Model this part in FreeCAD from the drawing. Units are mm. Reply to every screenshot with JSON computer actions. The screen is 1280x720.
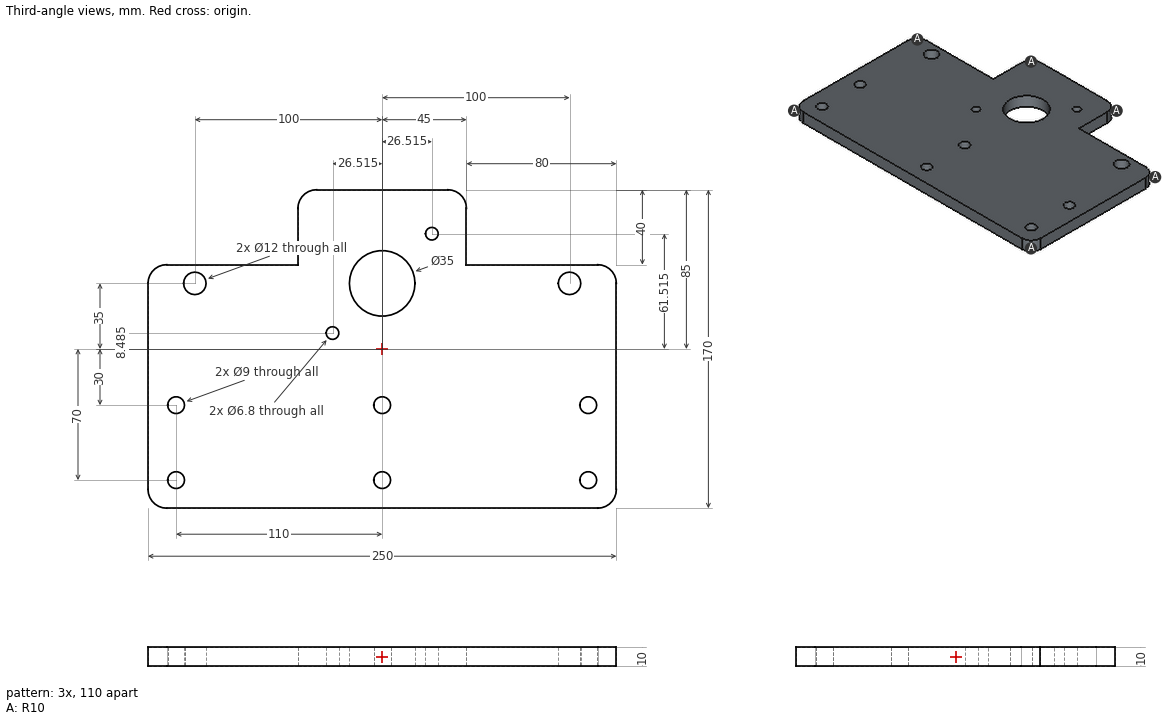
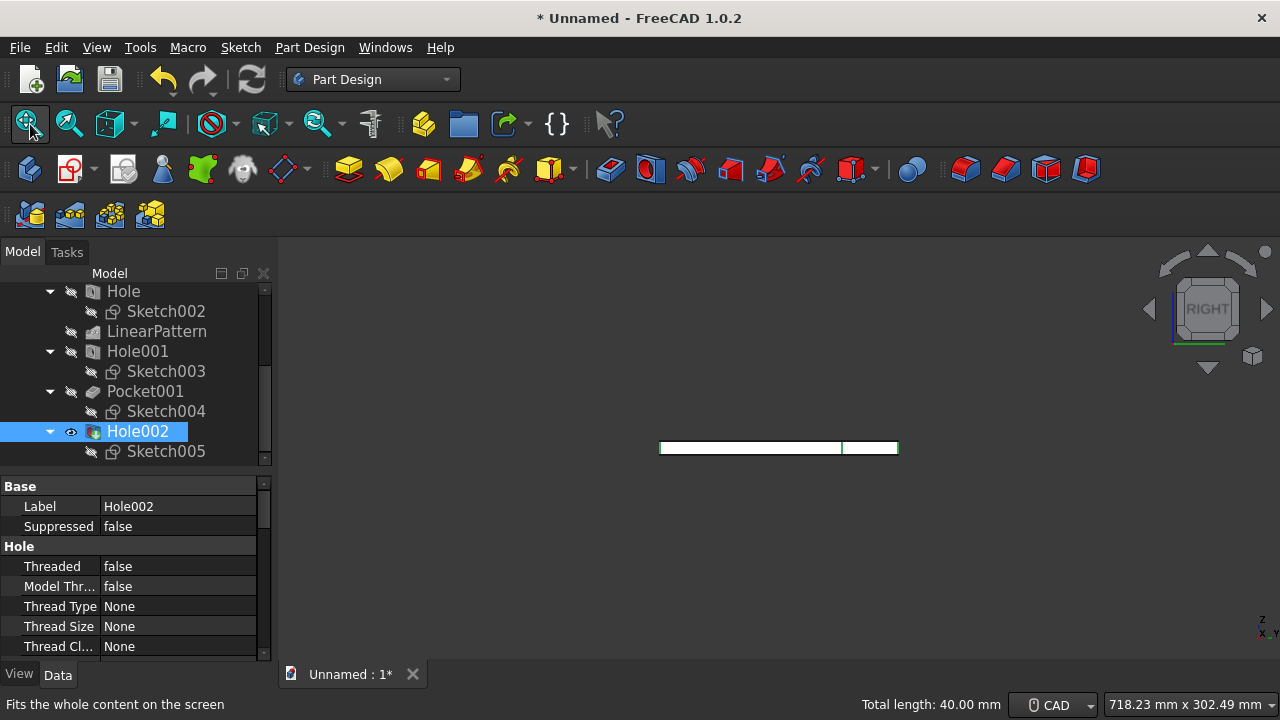
{"action": "key", "text": "5"}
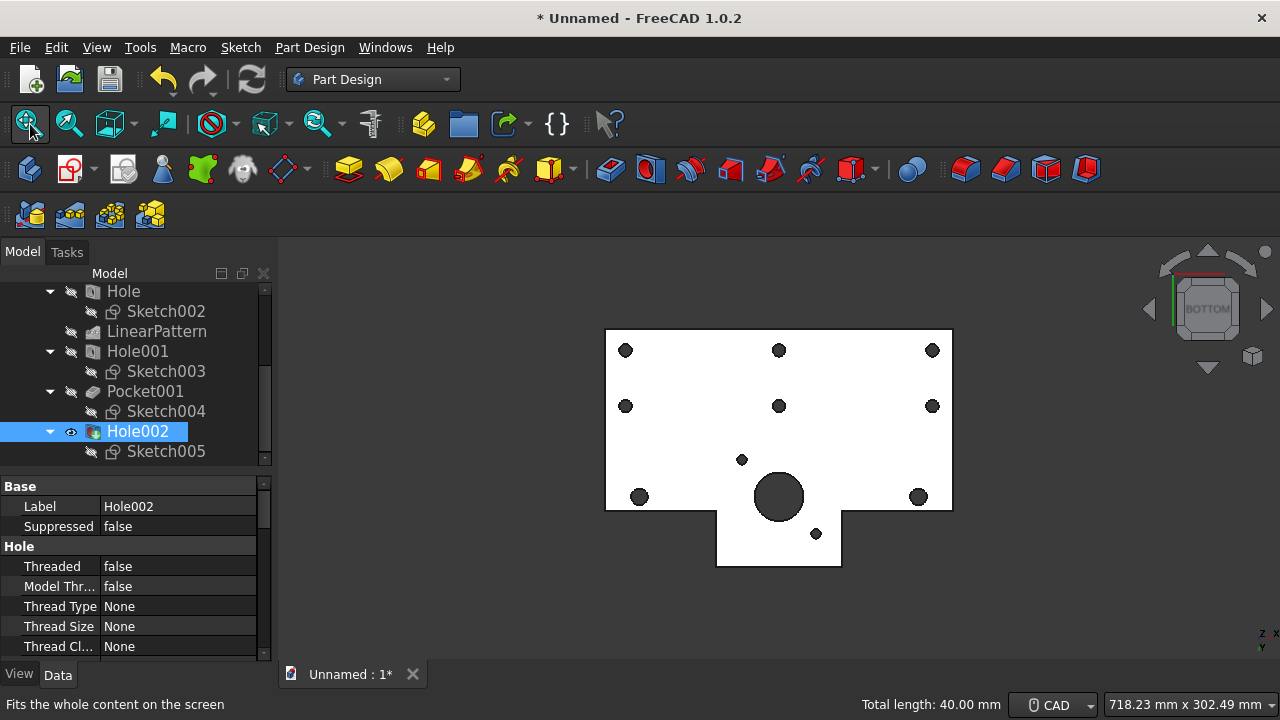
{"action": "scroll", "coordinate": [716, 566], "scroll_direction": "up", "scroll_amount": 6}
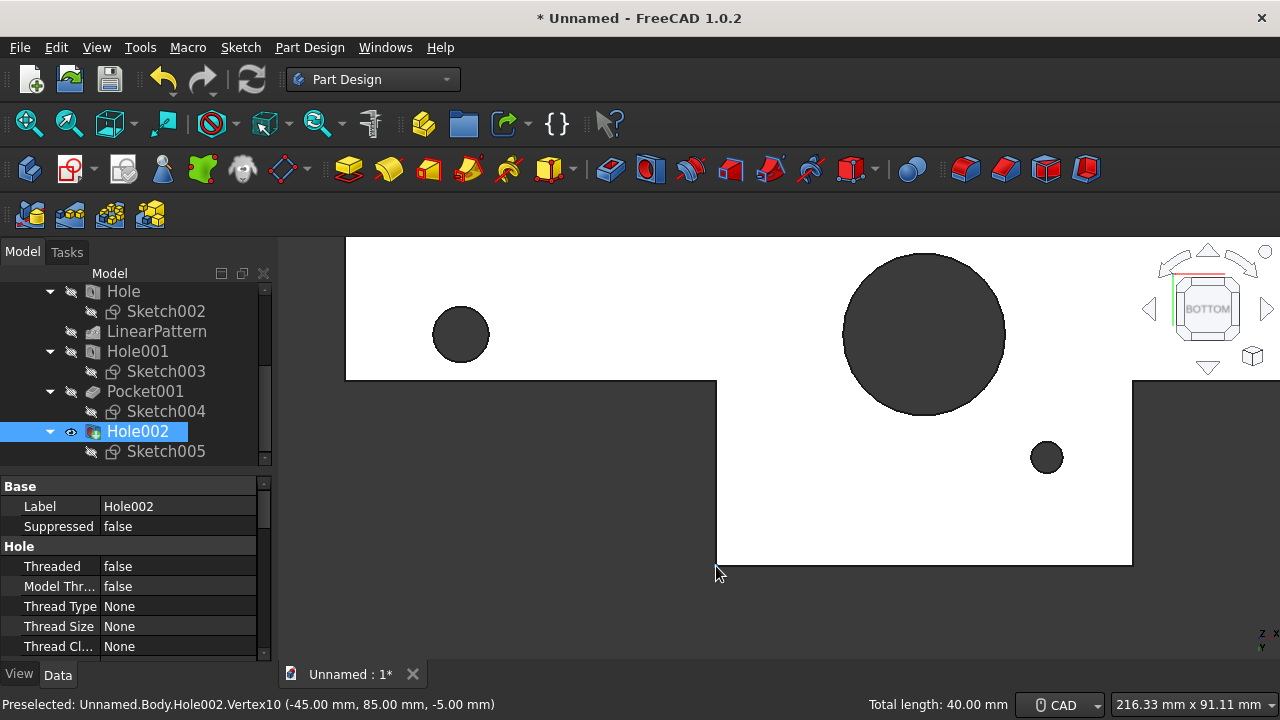
{"action": "left_click", "coordinate": [30, 124]}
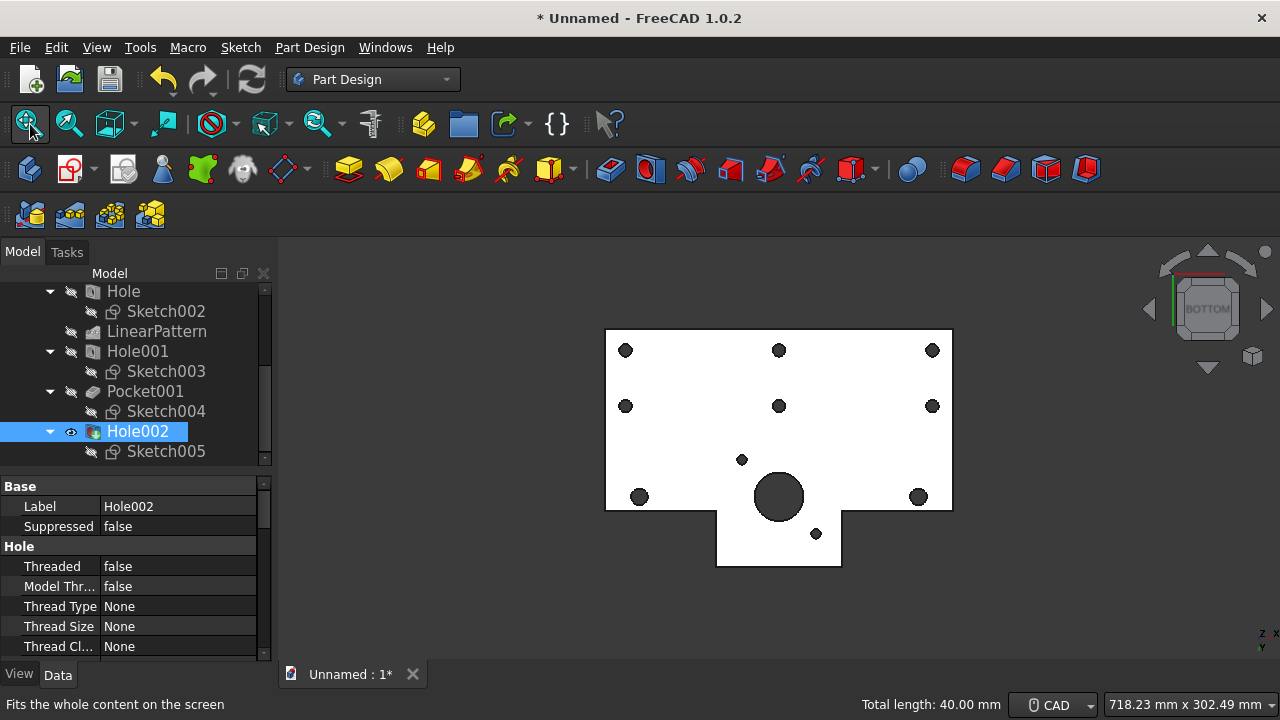
{"action": "key", "text": "4"}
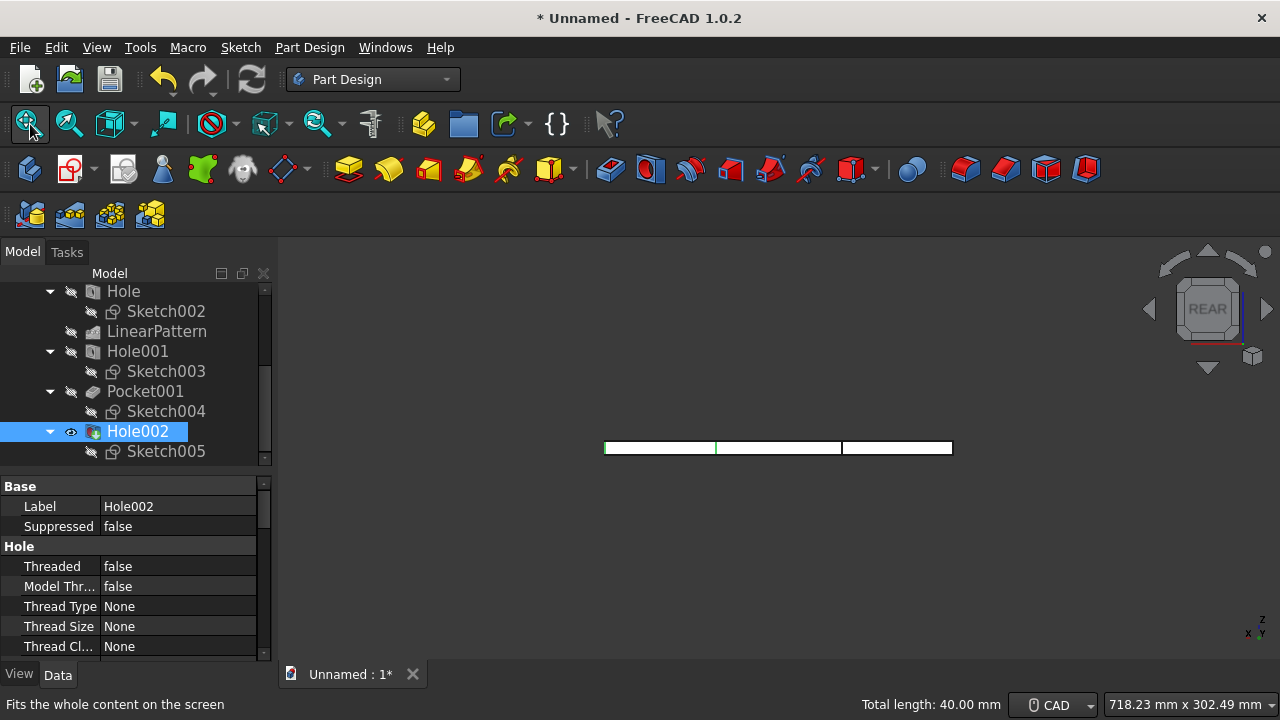
{"action": "left_click", "coordinate": [30, 124]}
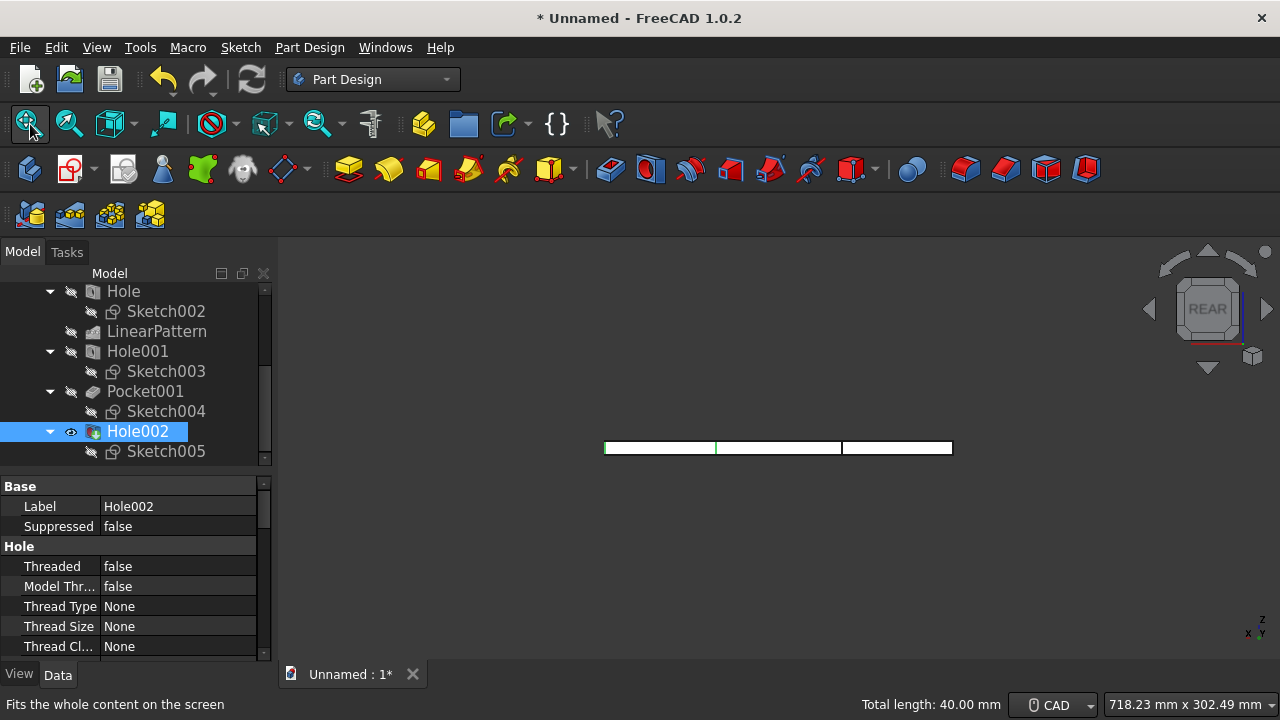
{"action": "left_click", "coordinate": [842, 447], "text": "ctrl"}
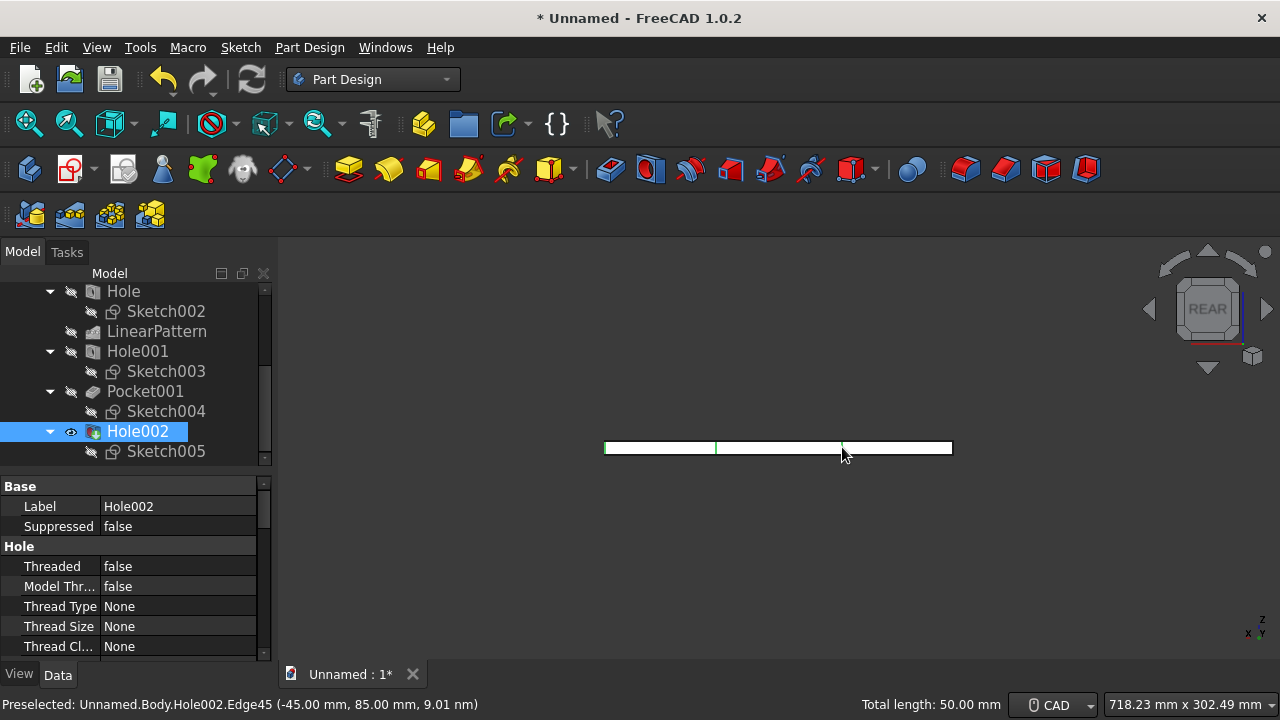
{"action": "left_click", "coordinate": [953, 447], "text": "ctrl"}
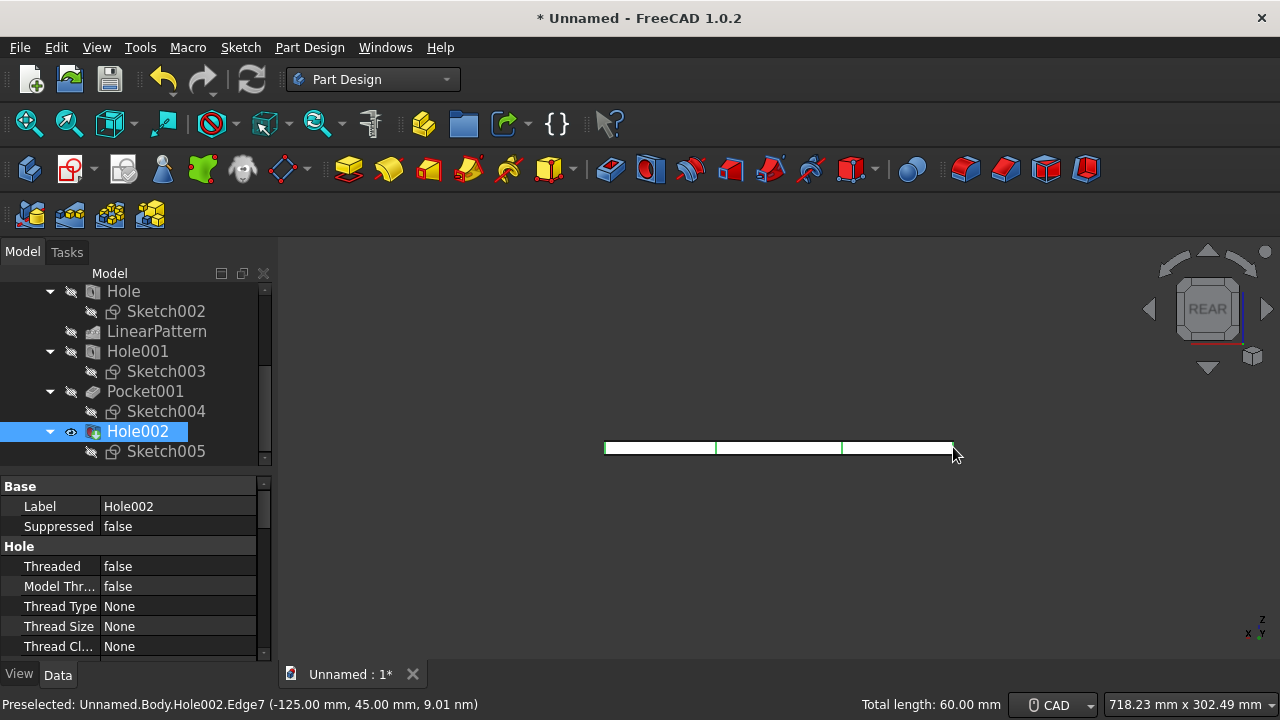
{"action": "left_click", "coordinate": [966, 170]}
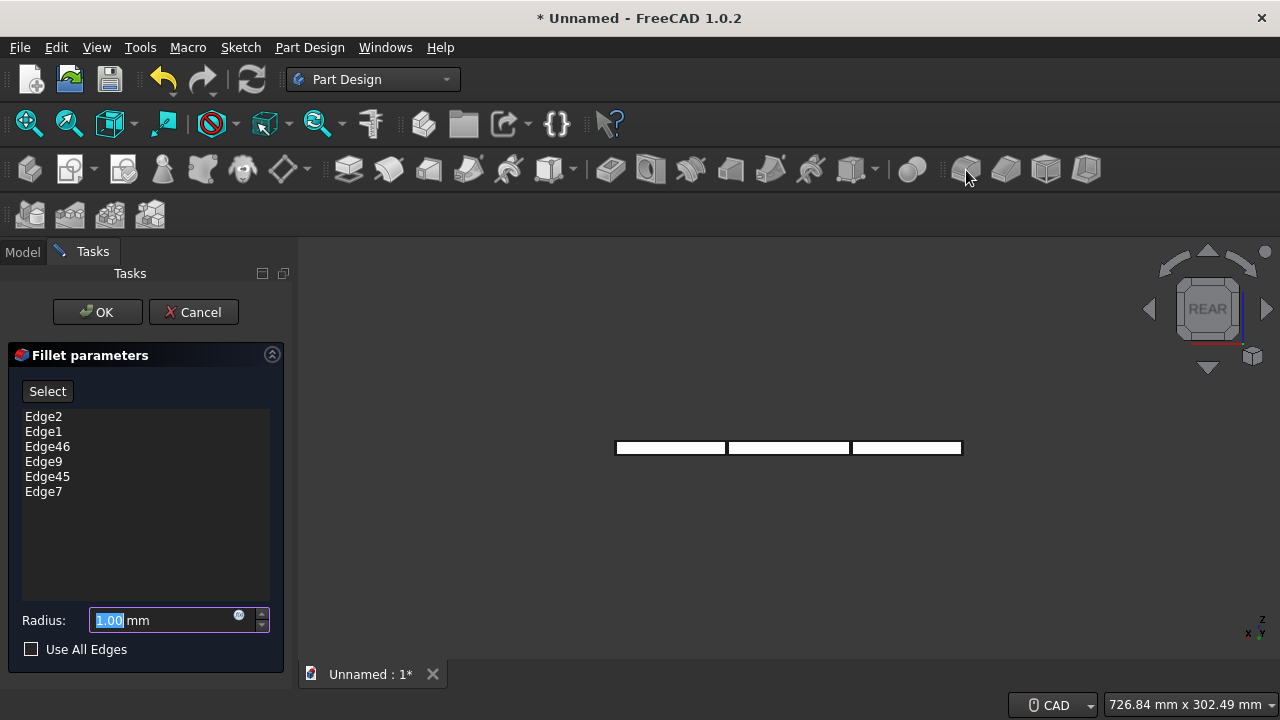
{"action": "type", "text": "10"}
{"action": "key", "text": "Tab"}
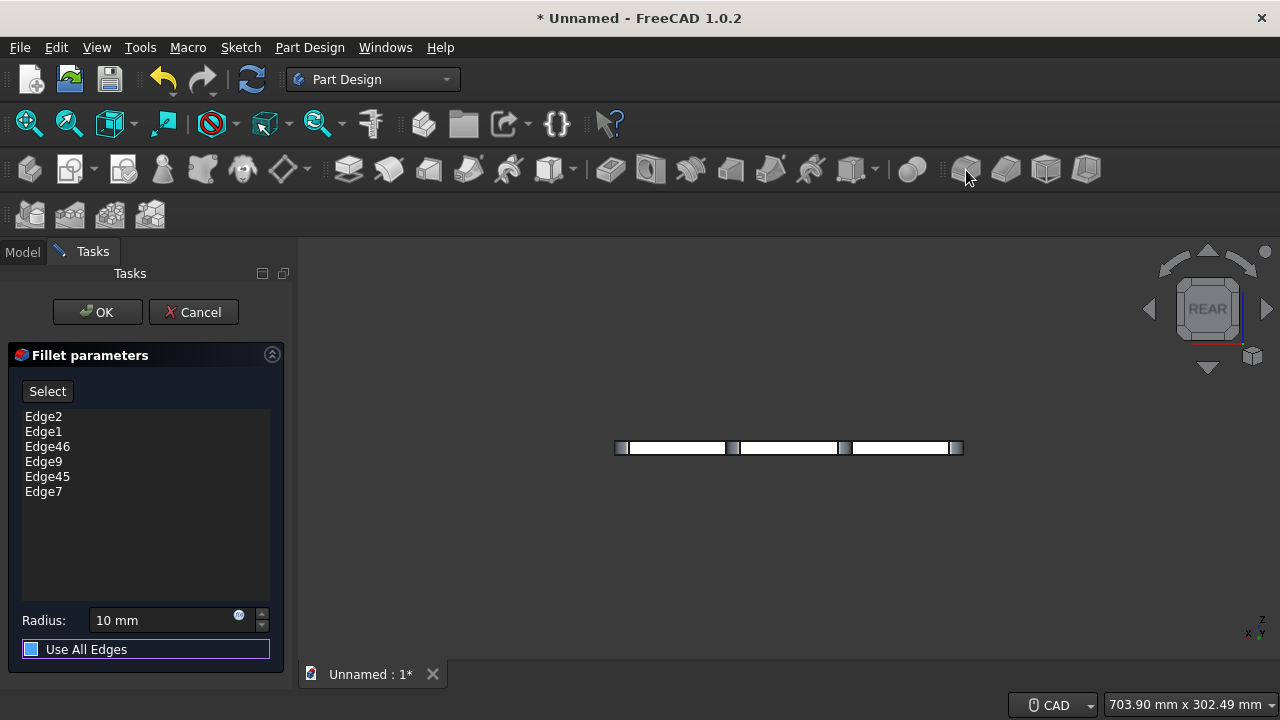
{"action": "left_click", "coordinate": [98, 312]}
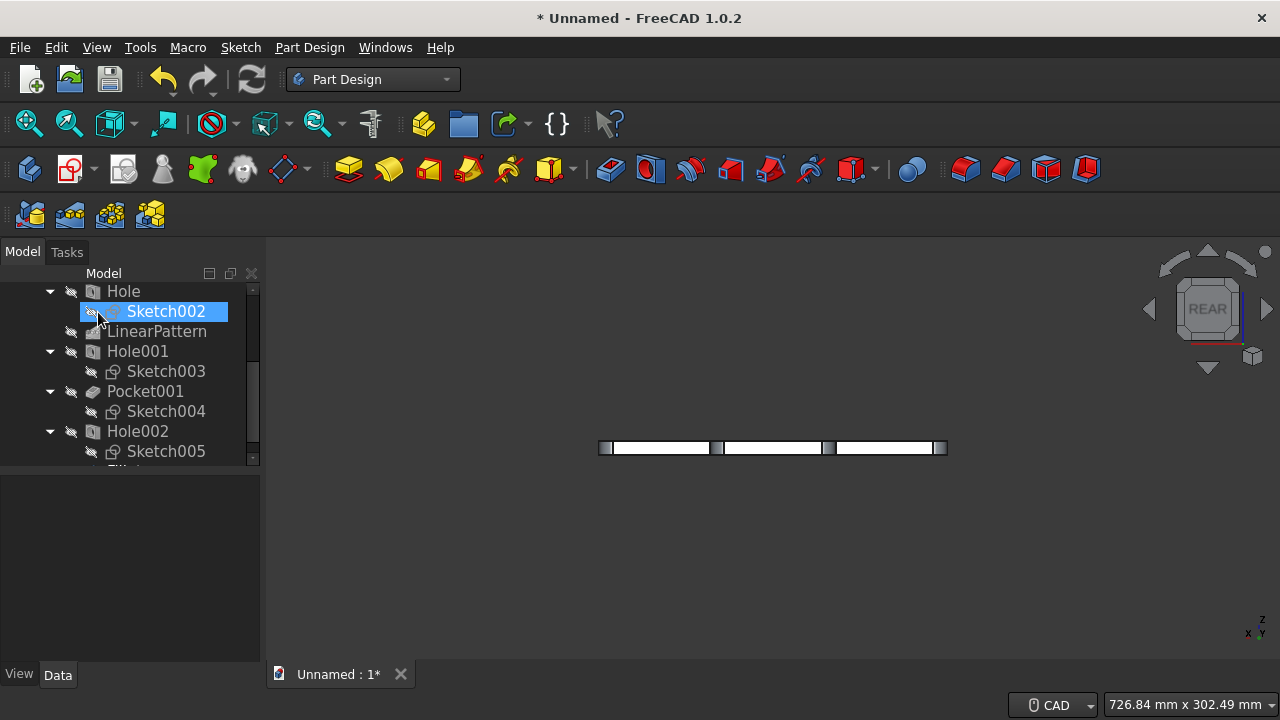
{"action": "key", "text": "0"}